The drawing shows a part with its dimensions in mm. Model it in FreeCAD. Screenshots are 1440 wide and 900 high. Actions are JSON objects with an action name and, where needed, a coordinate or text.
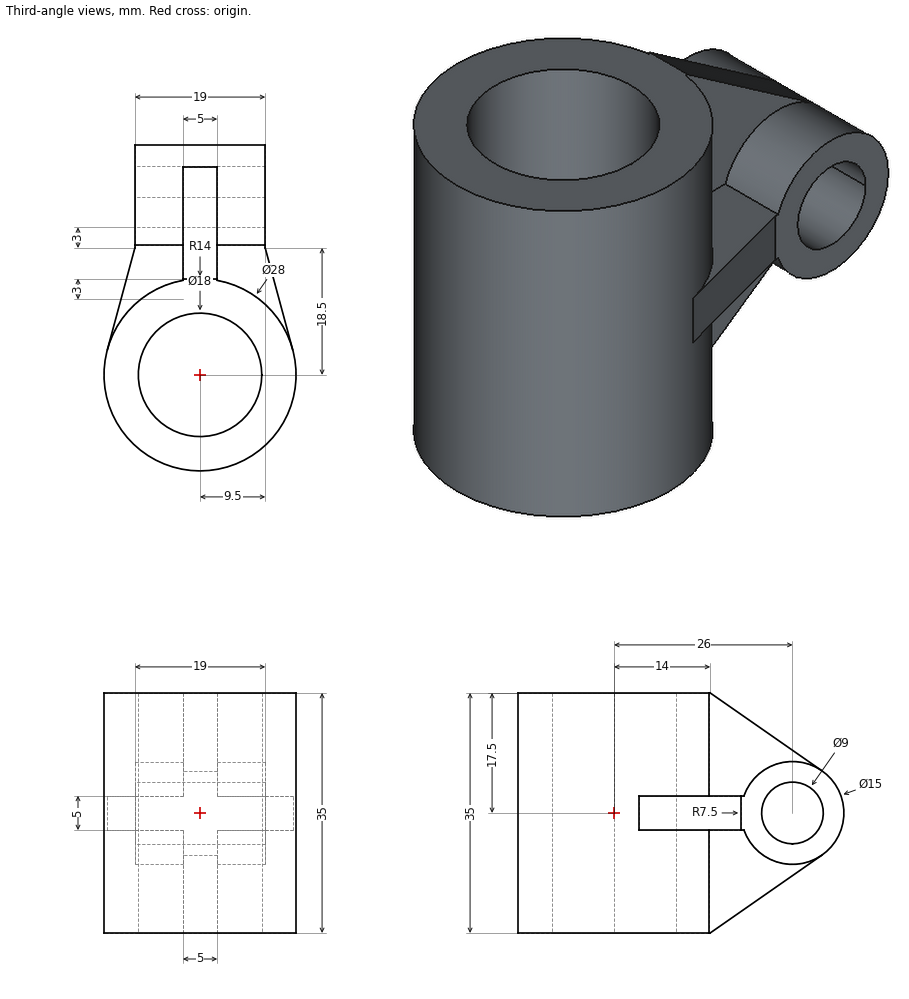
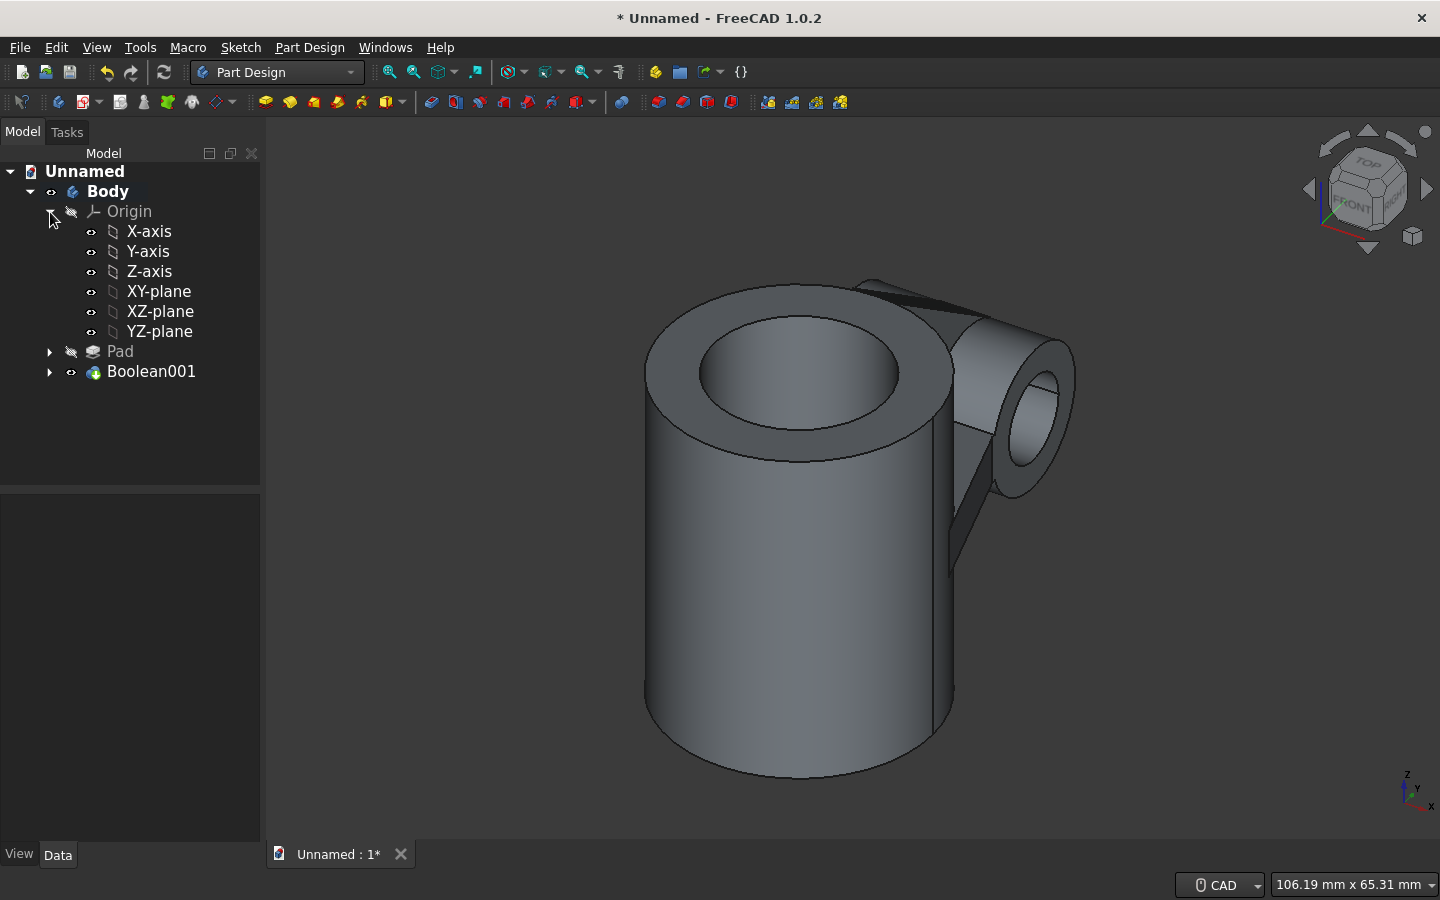
{"action": "left_click", "coordinate": [136, 312]}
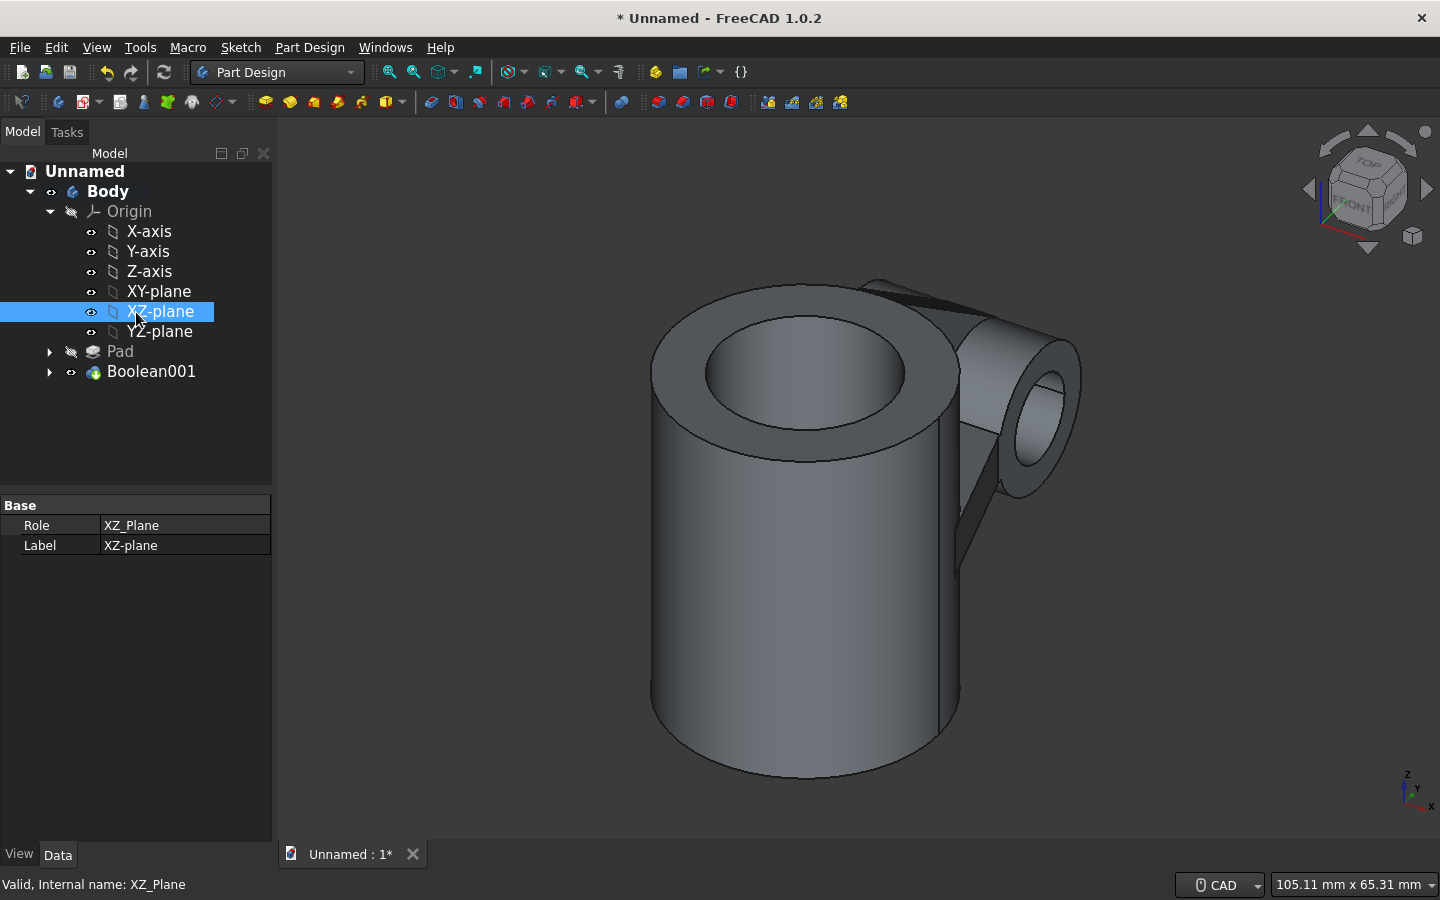
{"action": "left_click", "coordinate": [216, 102]}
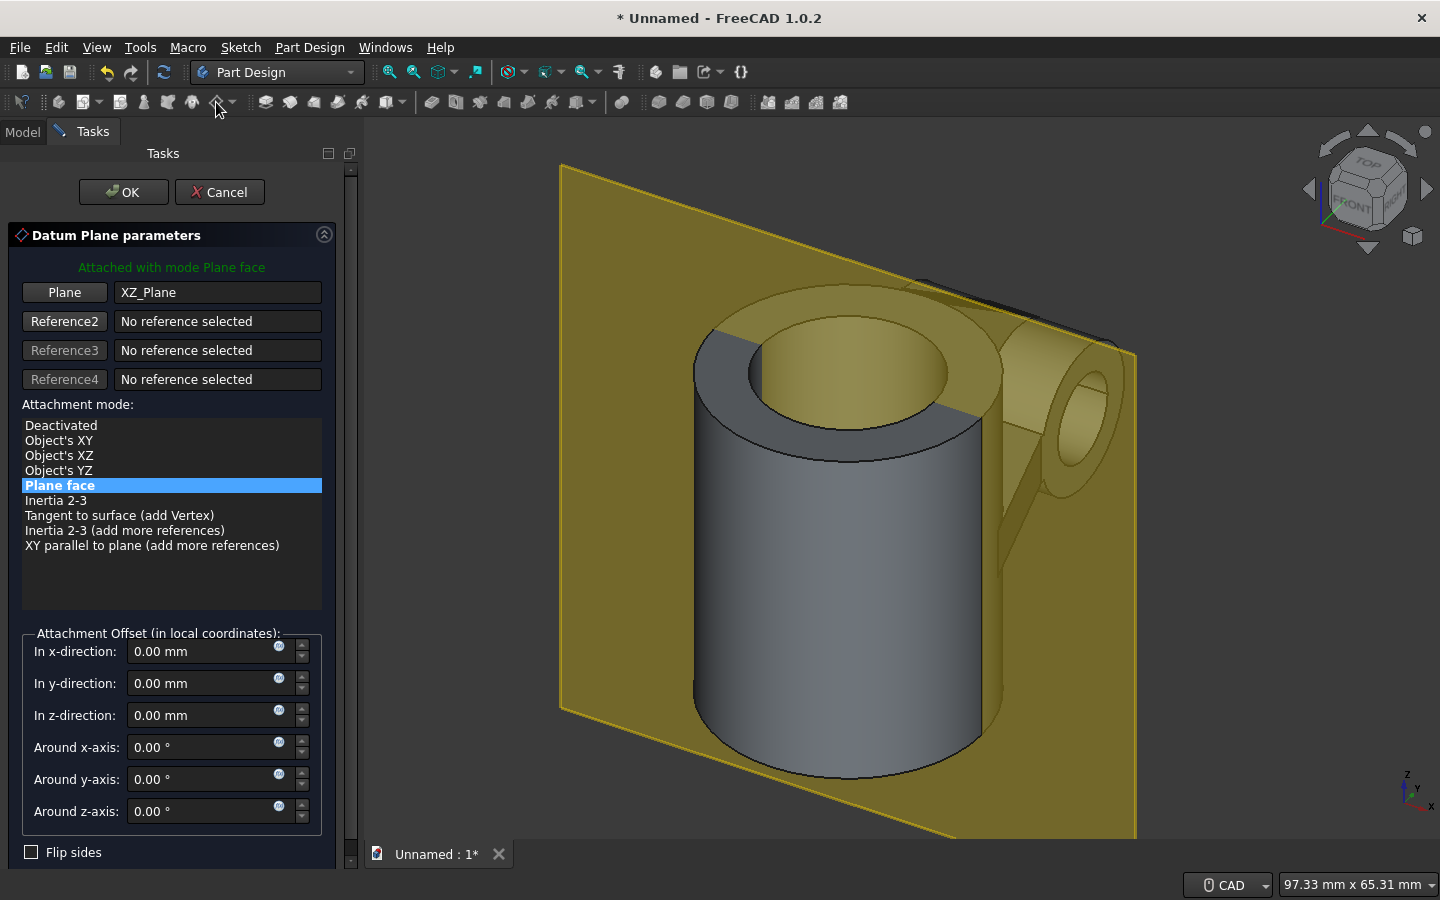
{"action": "triple_click", "coordinate": [210, 715]}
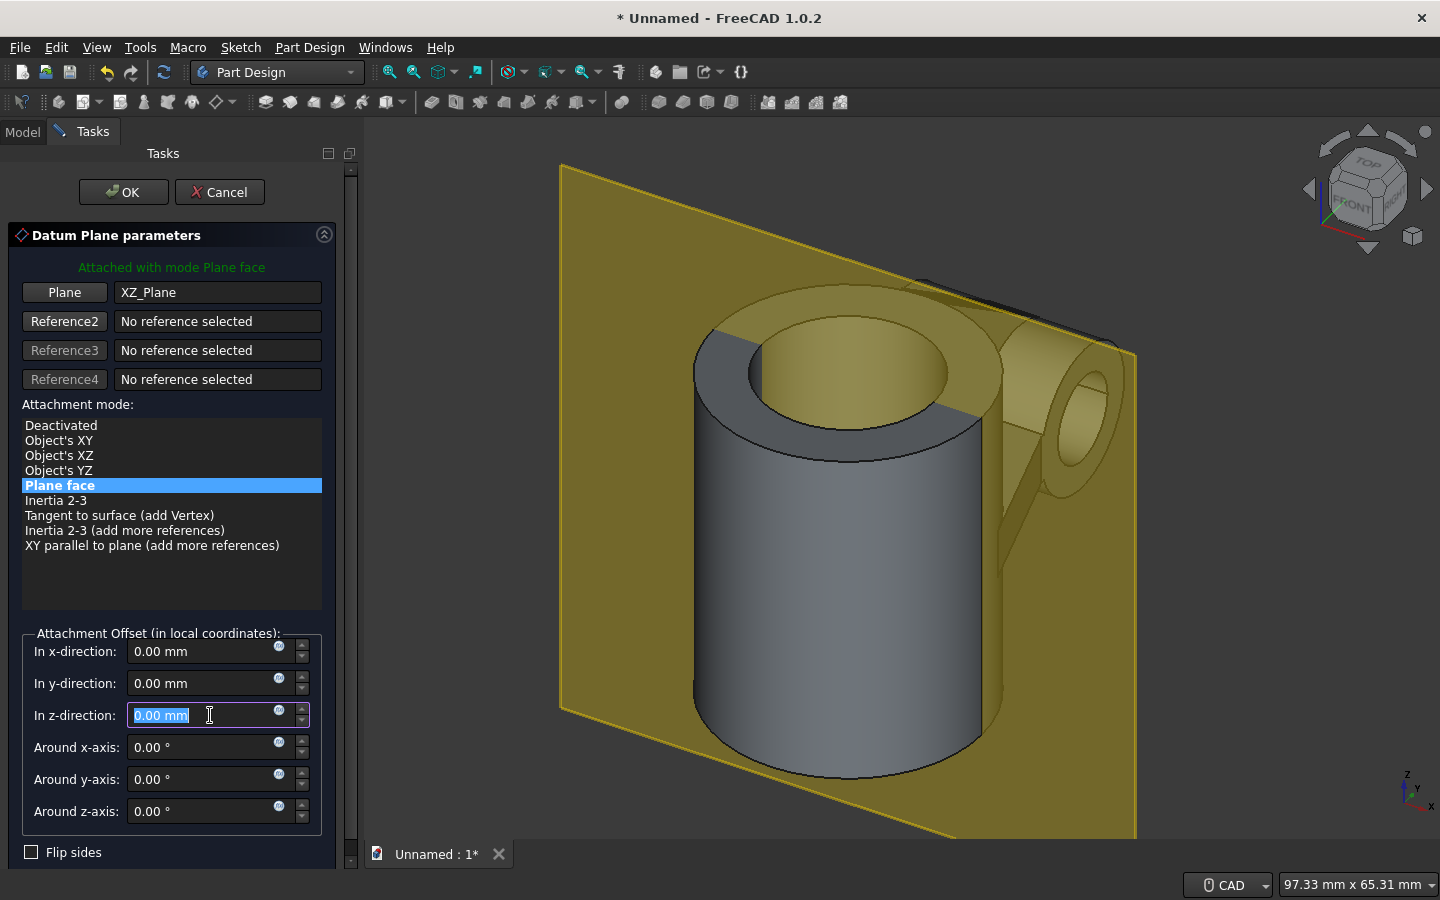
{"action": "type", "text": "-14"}
{"action": "key", "text": "Tab"}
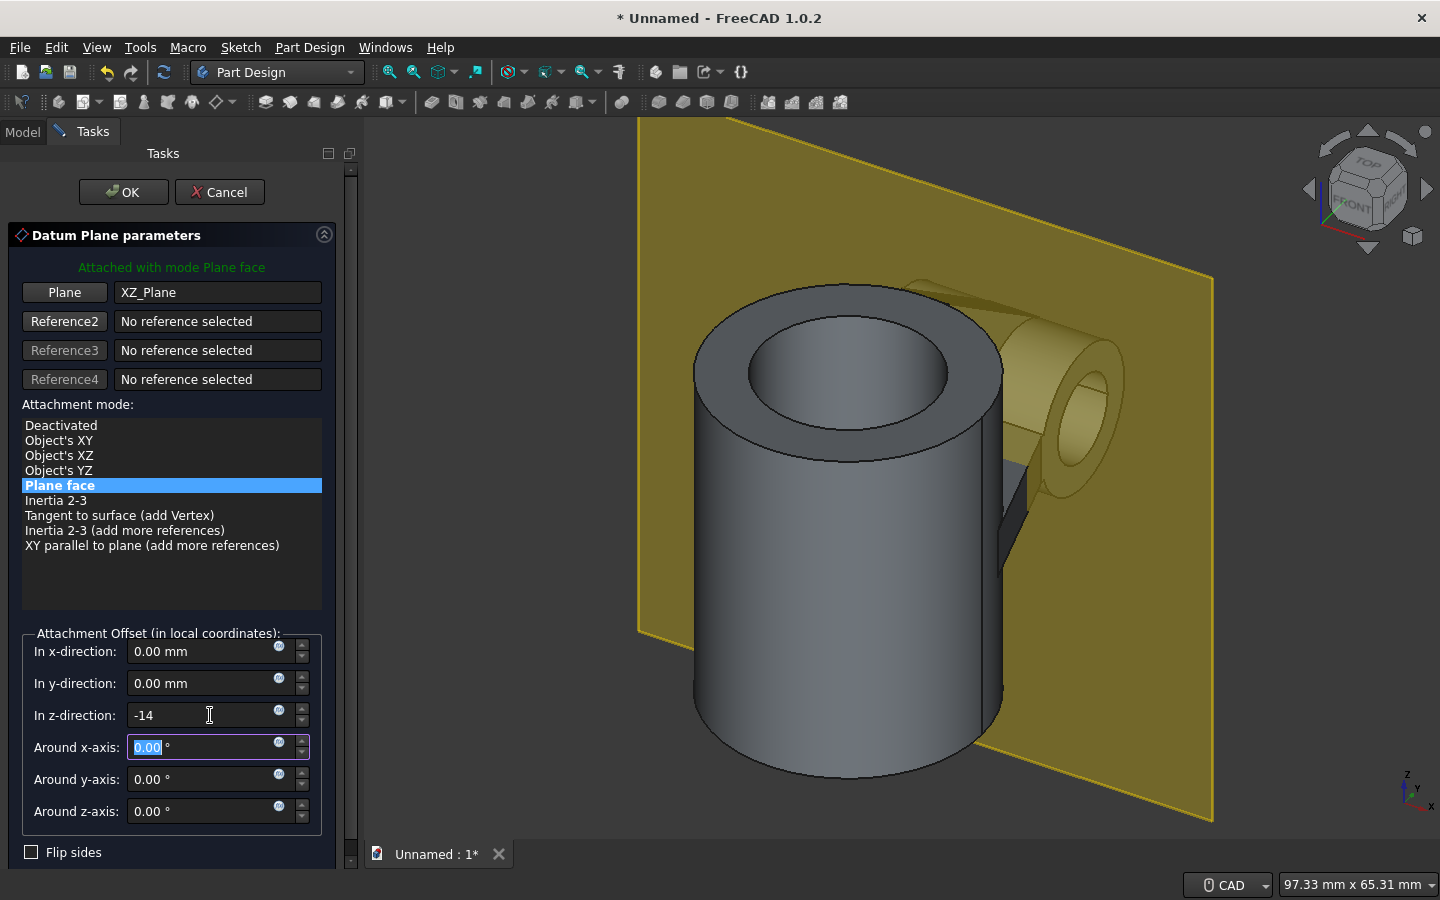
{"action": "left_click", "coordinate": [124, 192]}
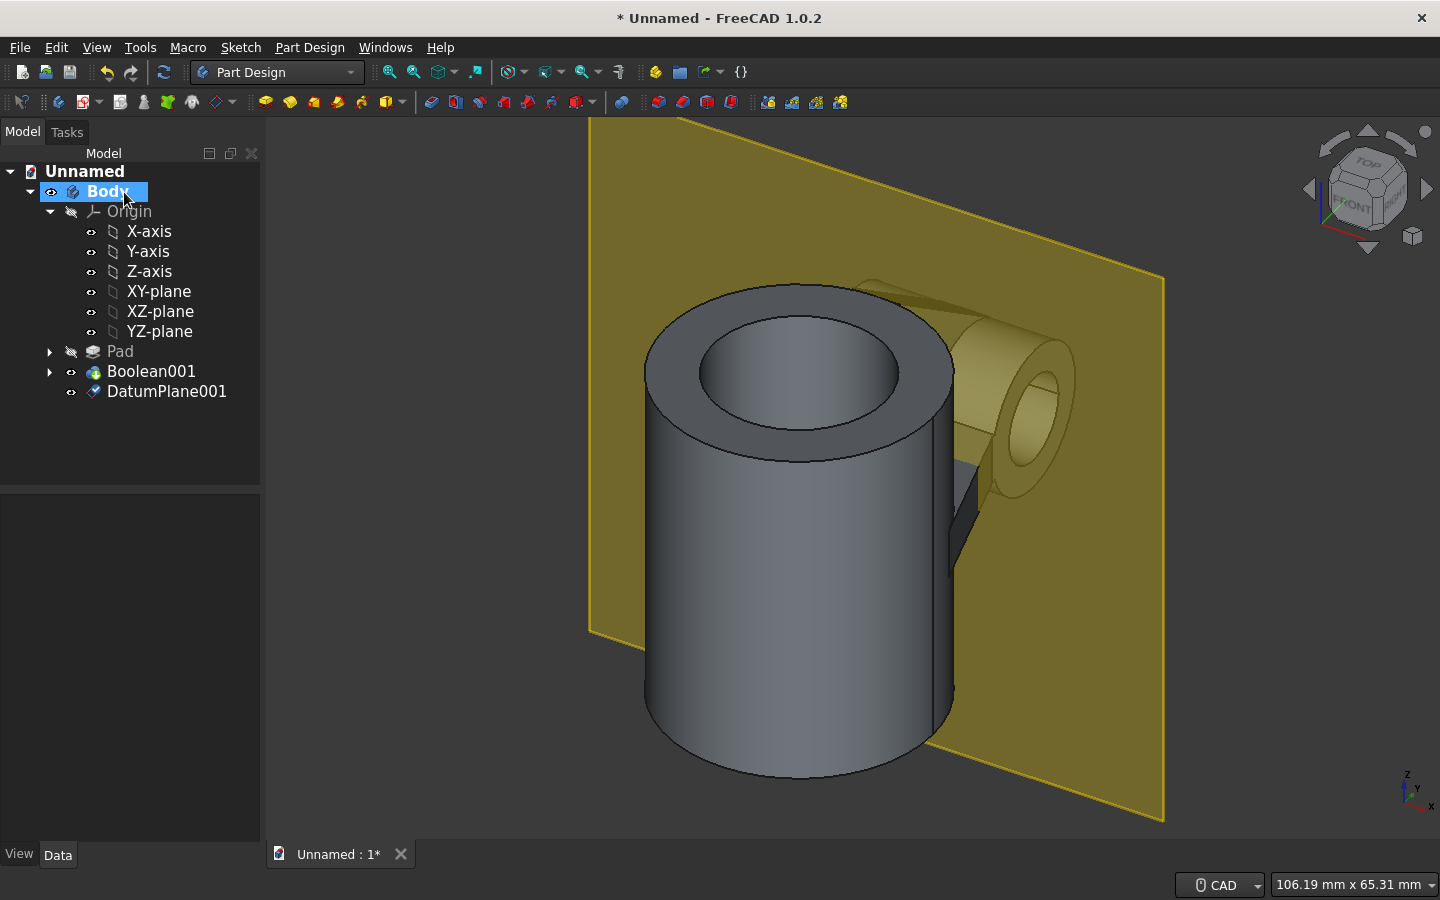
{"action": "left_click", "coordinate": [116, 392]}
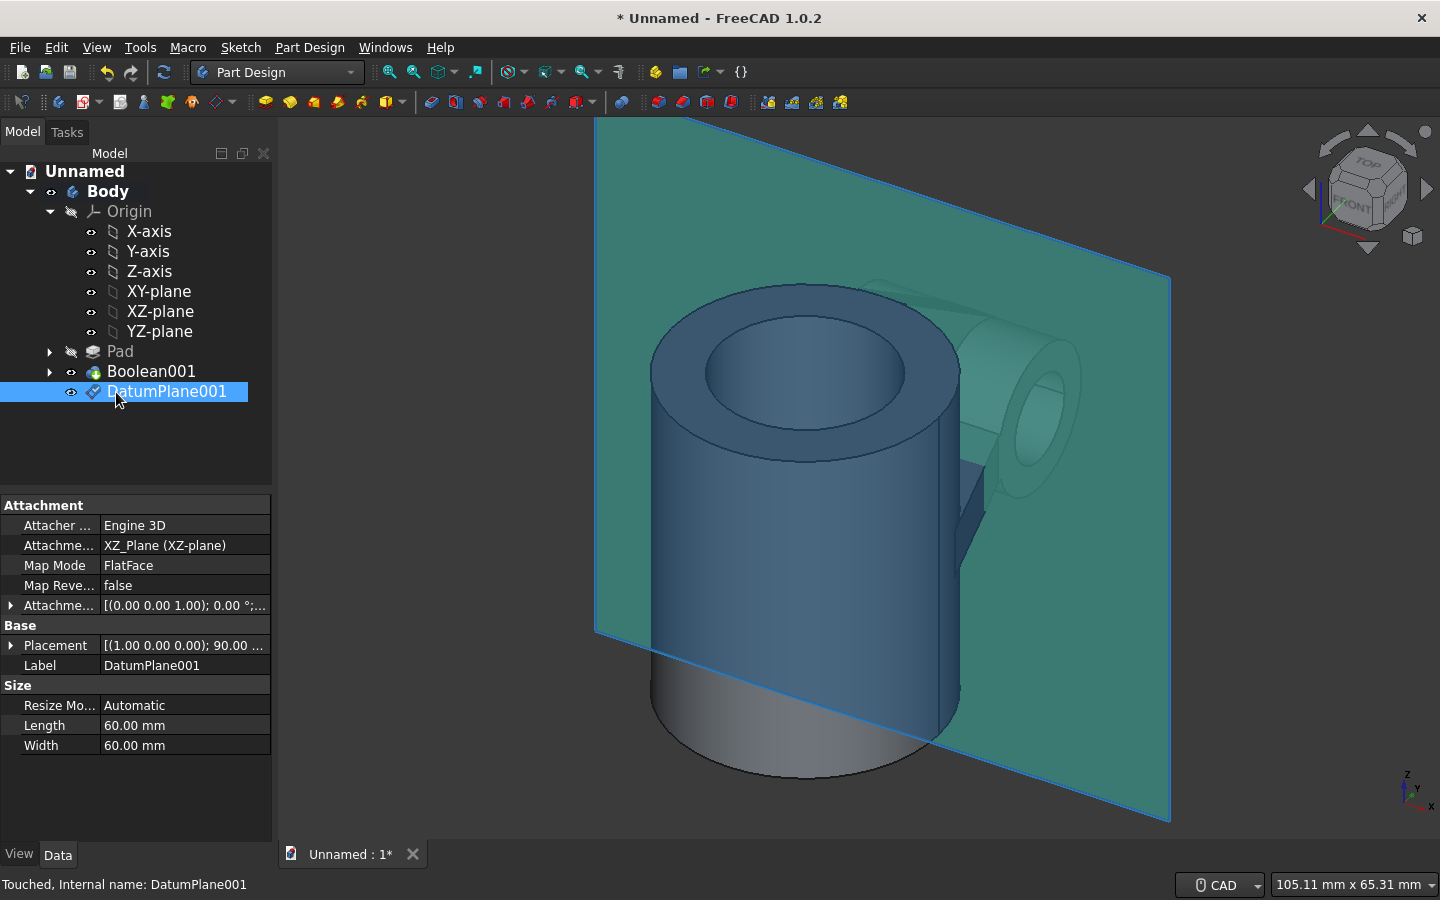
{"action": "left_click", "coordinate": [84, 102]}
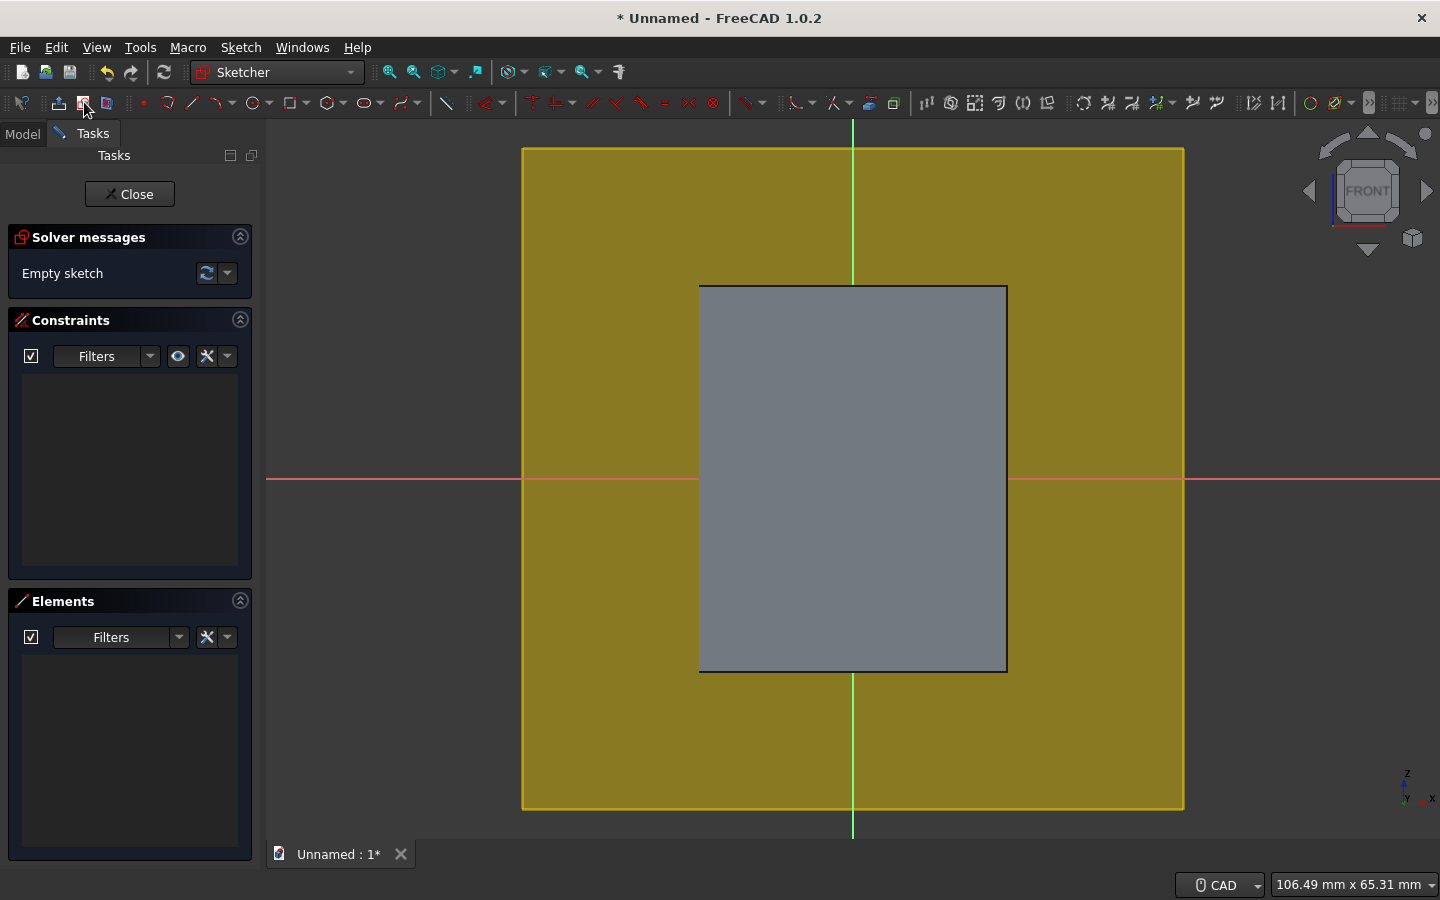
{"action": "key", "text": "q s"}